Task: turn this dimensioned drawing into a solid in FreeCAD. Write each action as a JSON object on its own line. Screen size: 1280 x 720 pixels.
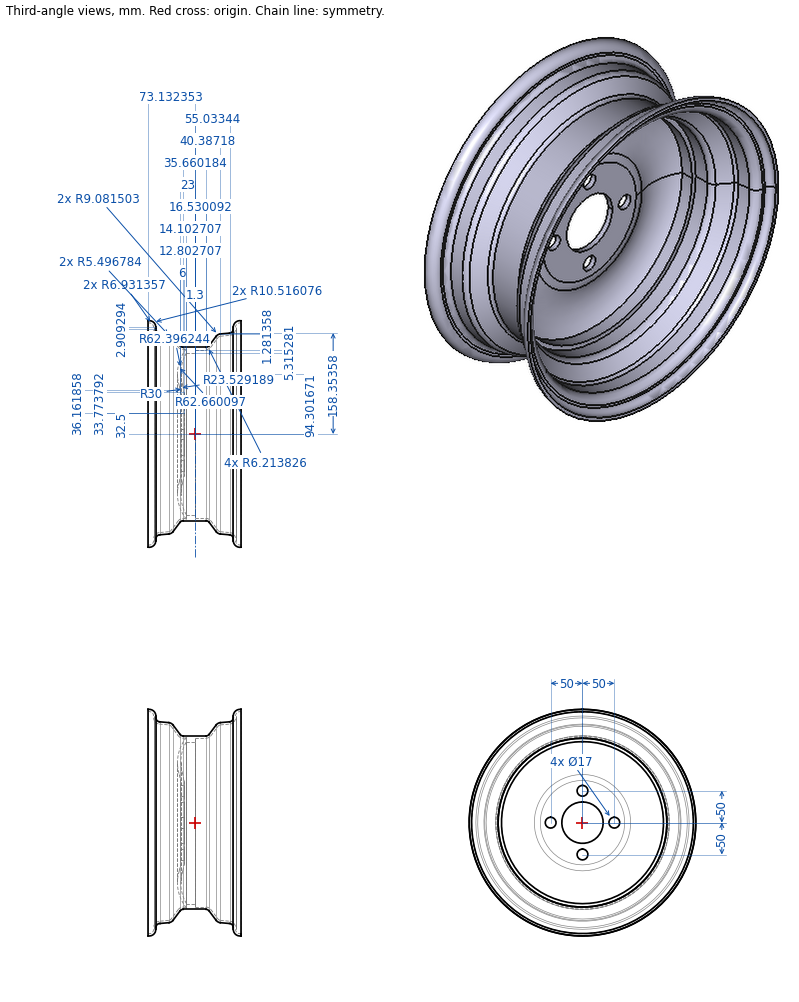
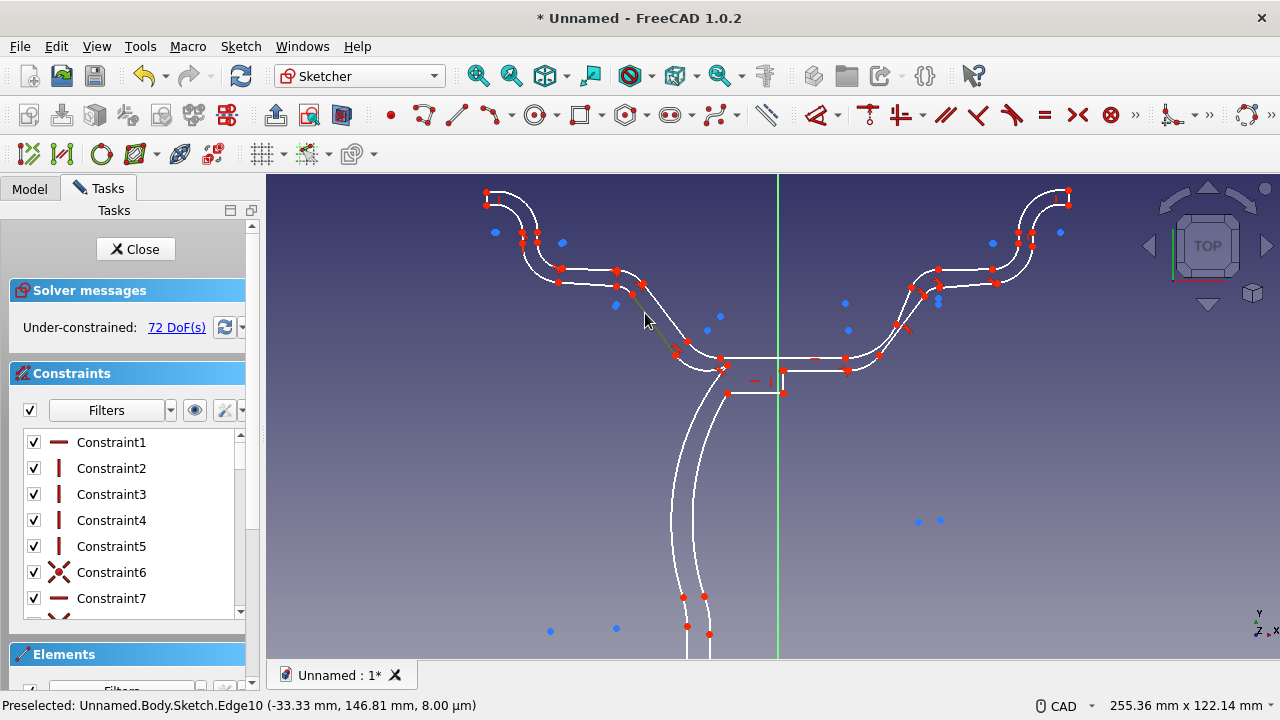
{"action": "left_click", "coordinate": [689, 366]}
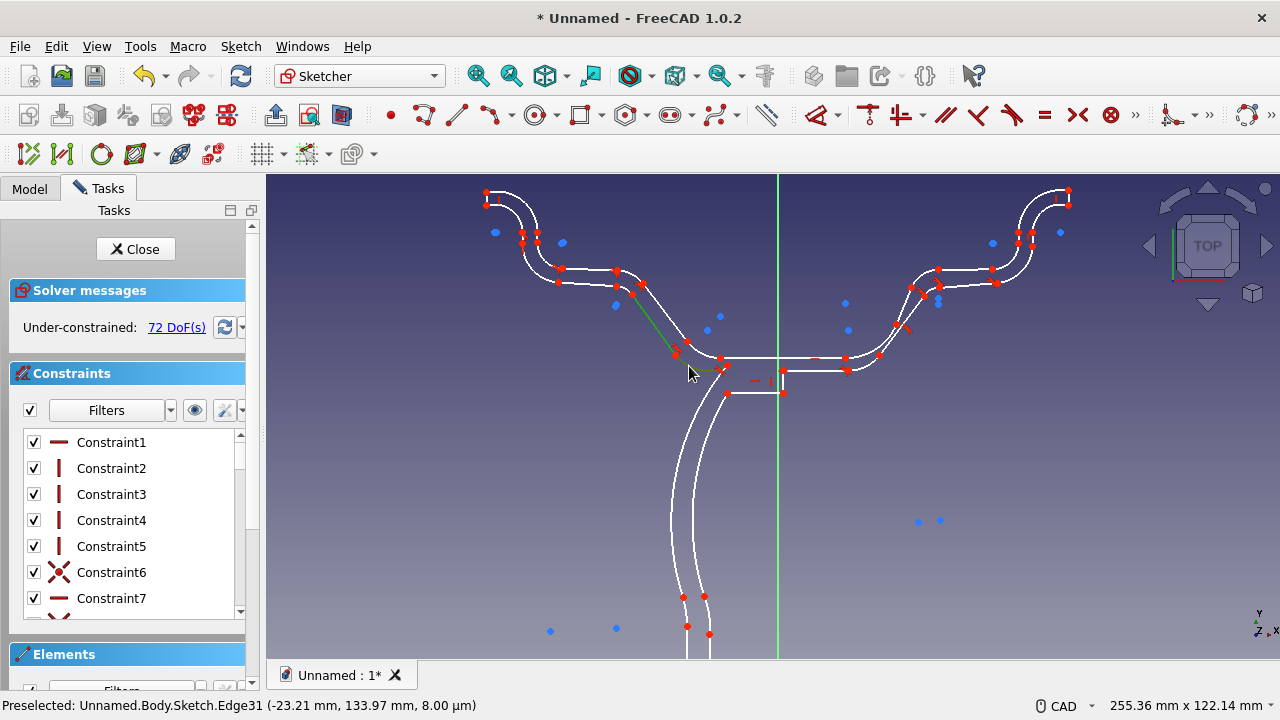
{"action": "key", "text": "t"}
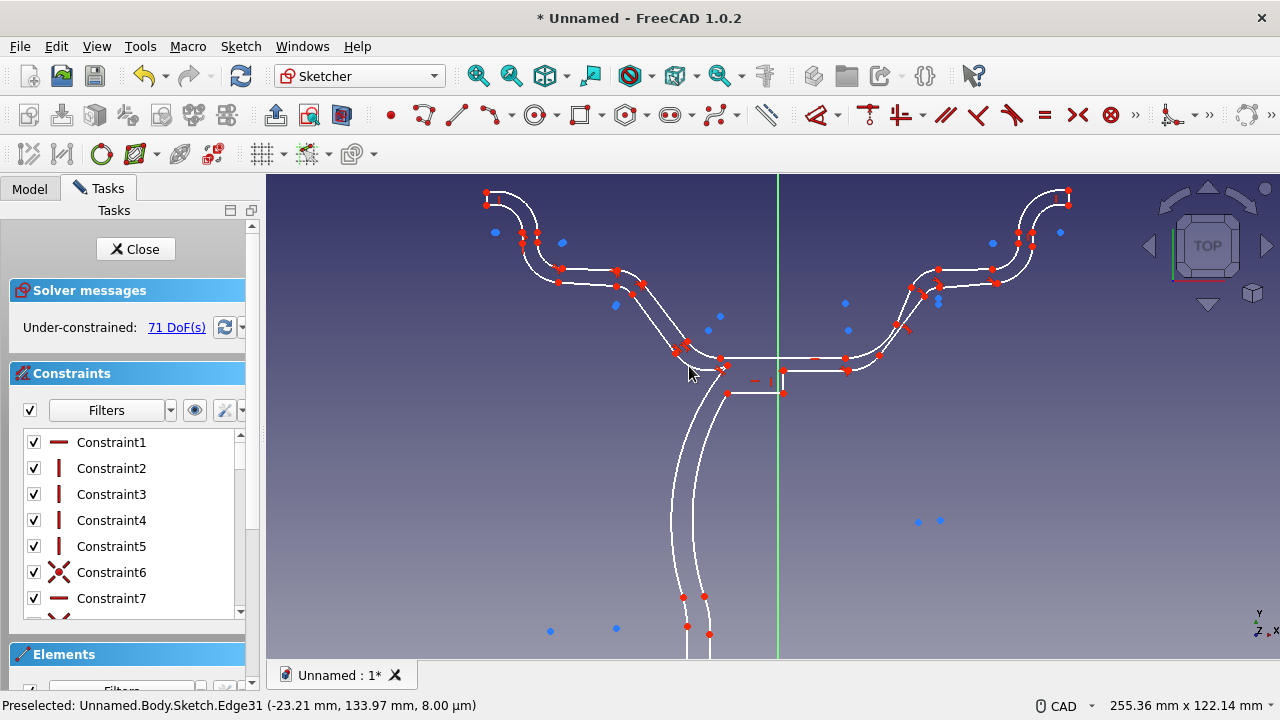
{"action": "scroll", "coordinate": [645, 313], "scroll_direction": "down", "scroll_amount": 4}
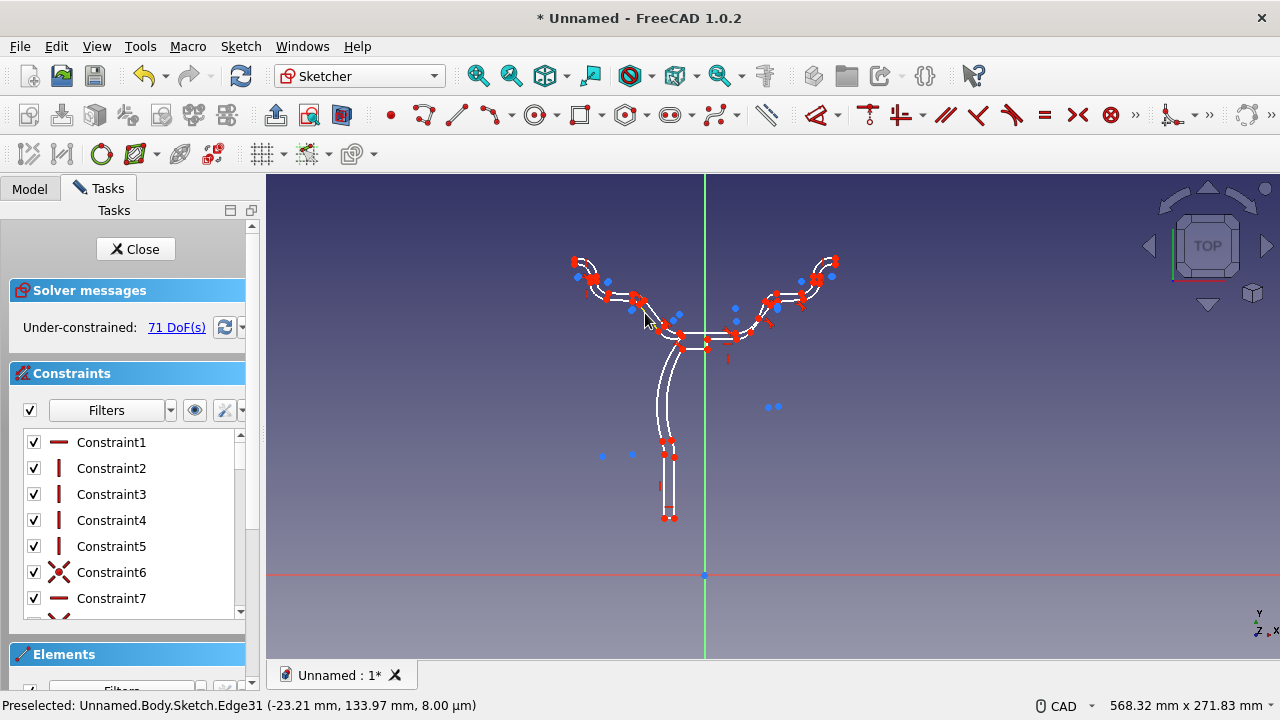
{"action": "scroll", "coordinate": [664, 473], "scroll_direction": "up", "scroll_amount": 2}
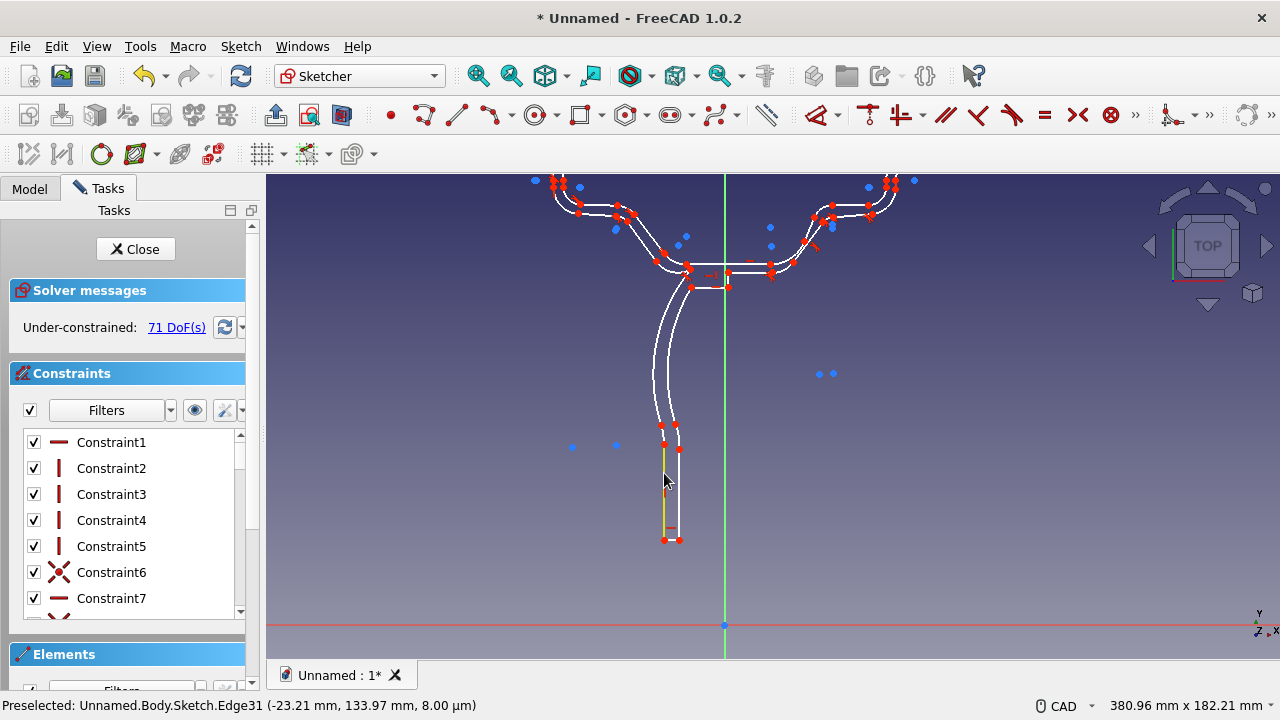
{"action": "left_click", "coordinate": [664, 473]}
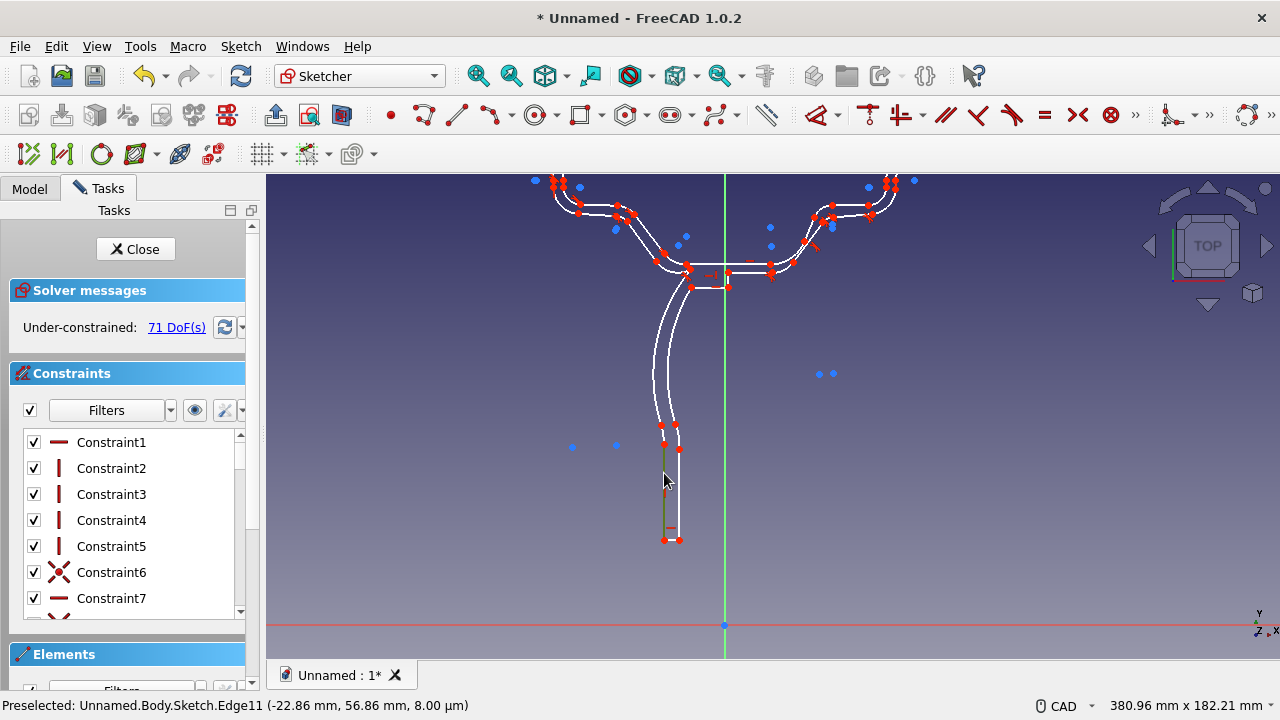
{"action": "scroll", "coordinate": [663, 435], "scroll_direction": "up", "scroll_amount": 2}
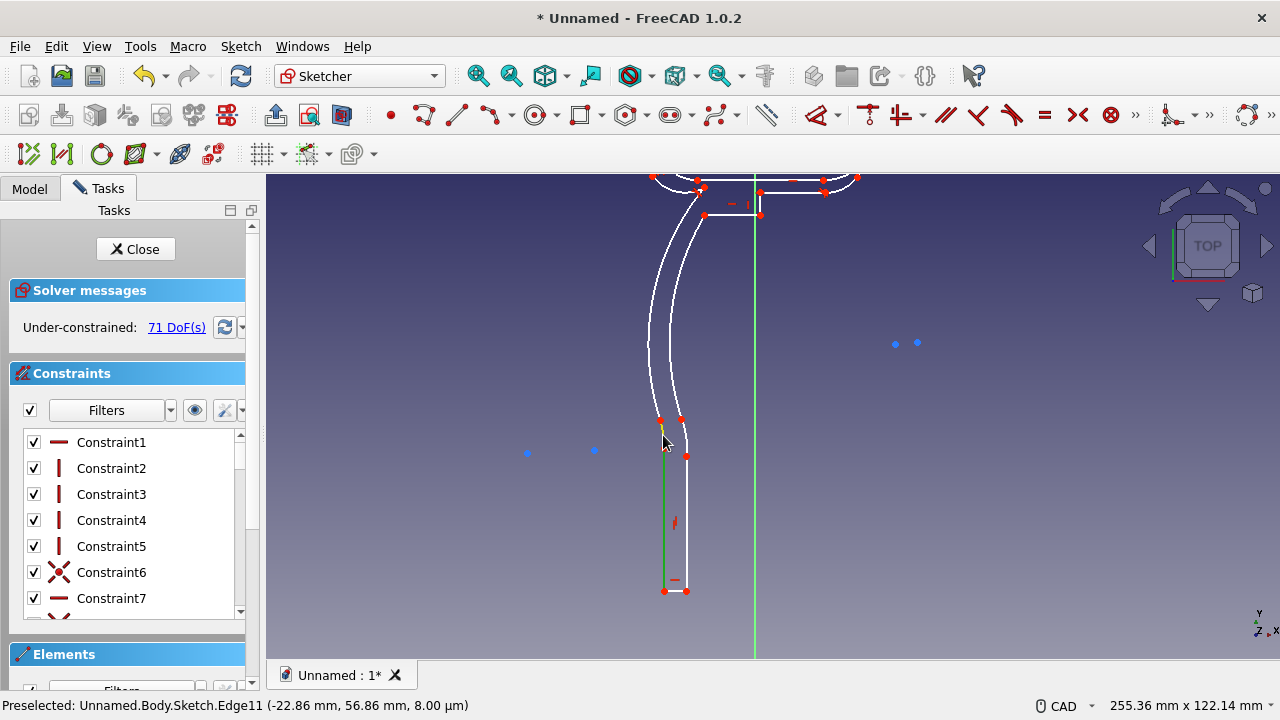
{"action": "left_click", "coordinate": [663, 434]}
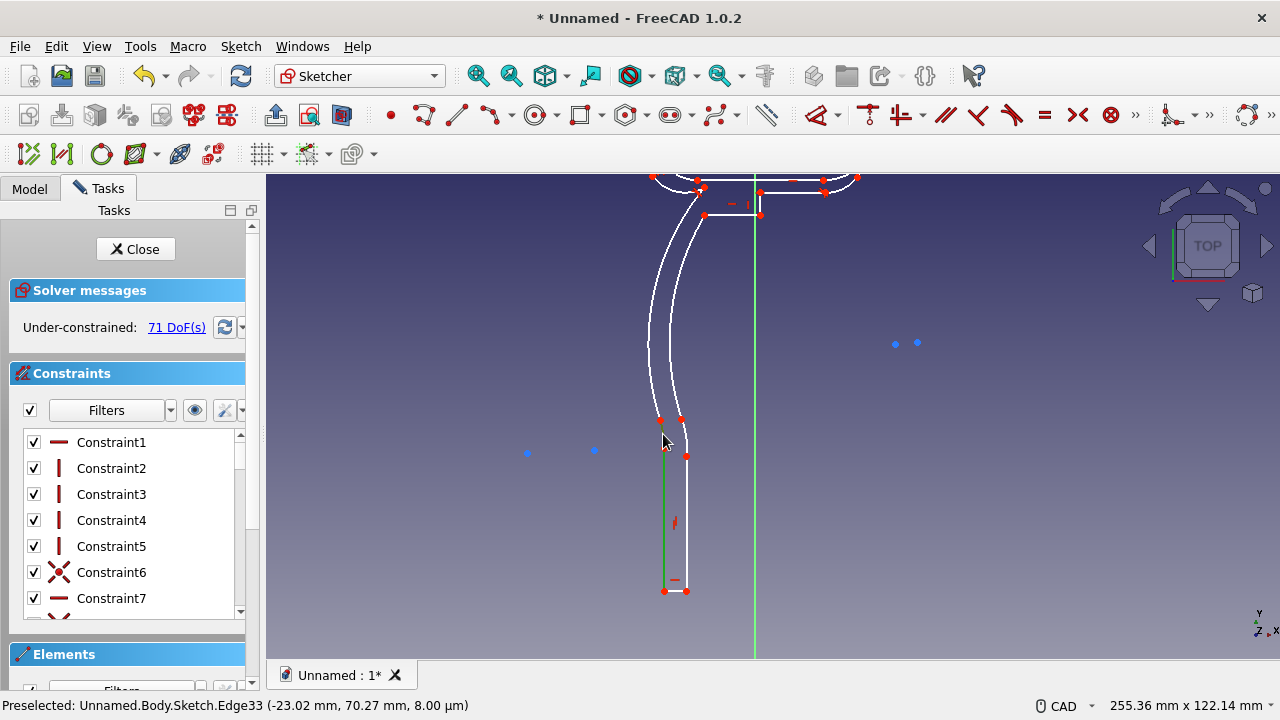
{"action": "left_click", "coordinate": [1012, 116]}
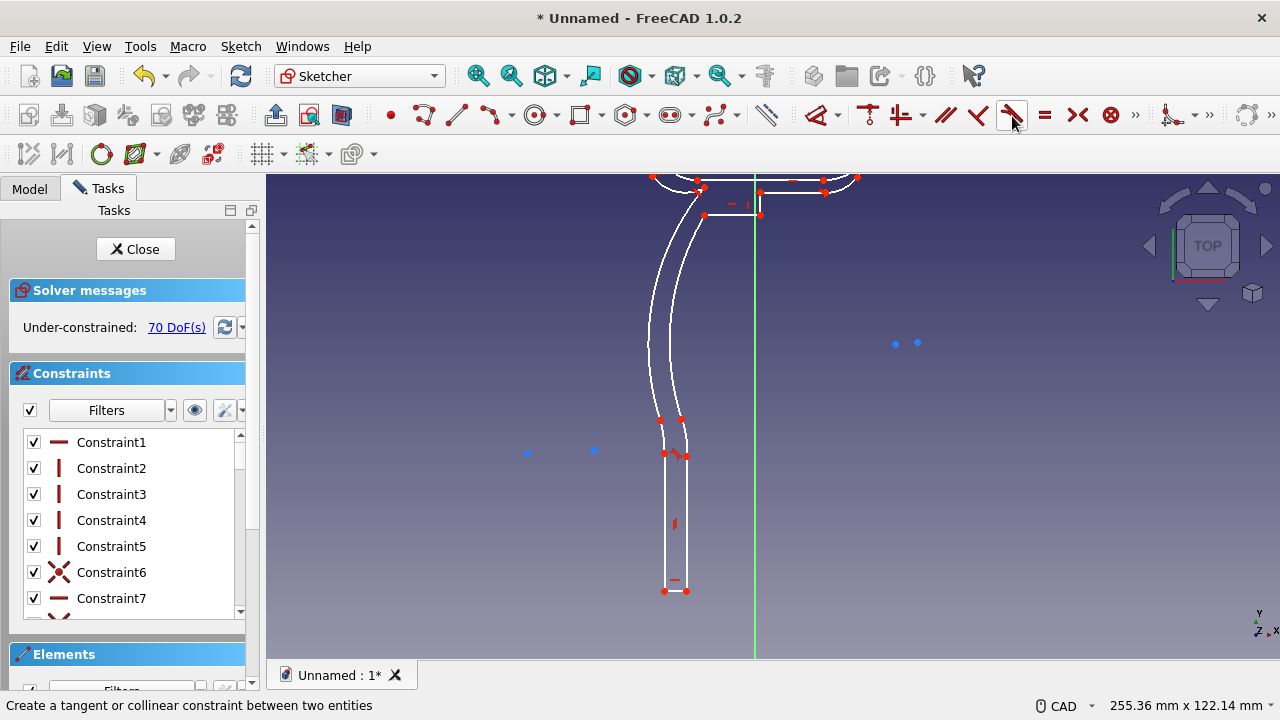
{"action": "left_click", "coordinate": [687, 551]}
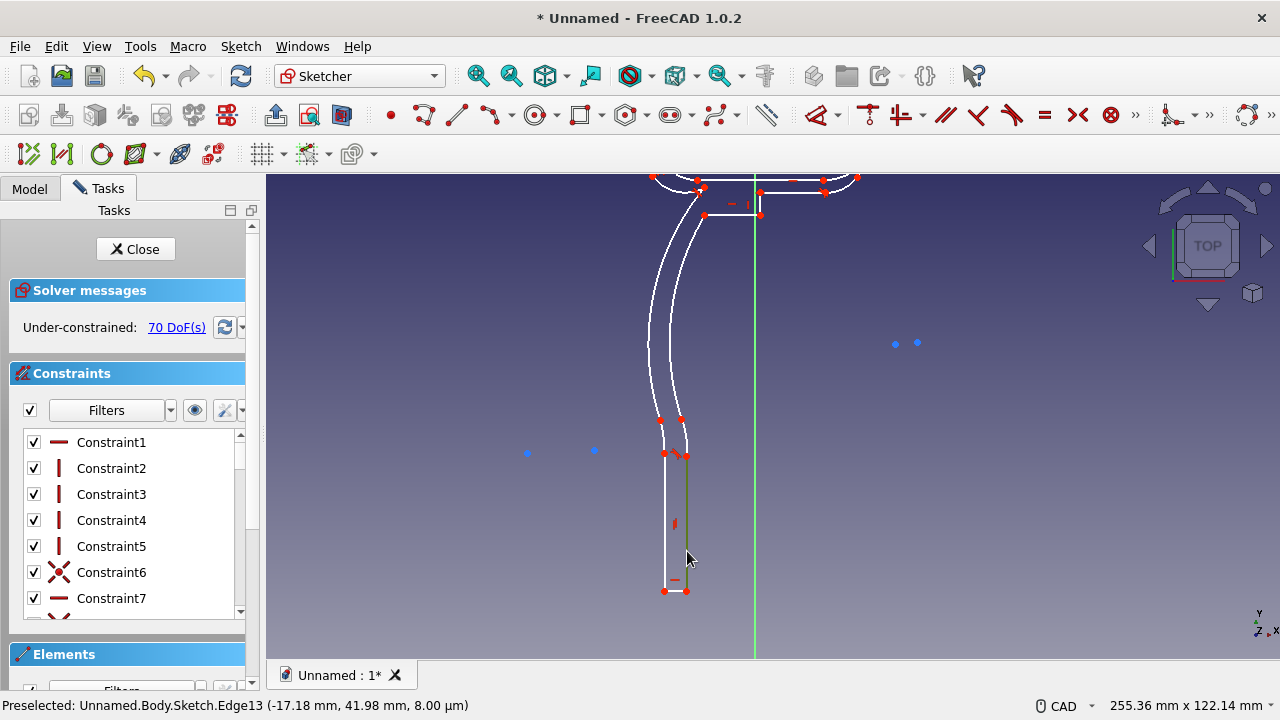
{"action": "left_click", "coordinate": [687, 445]}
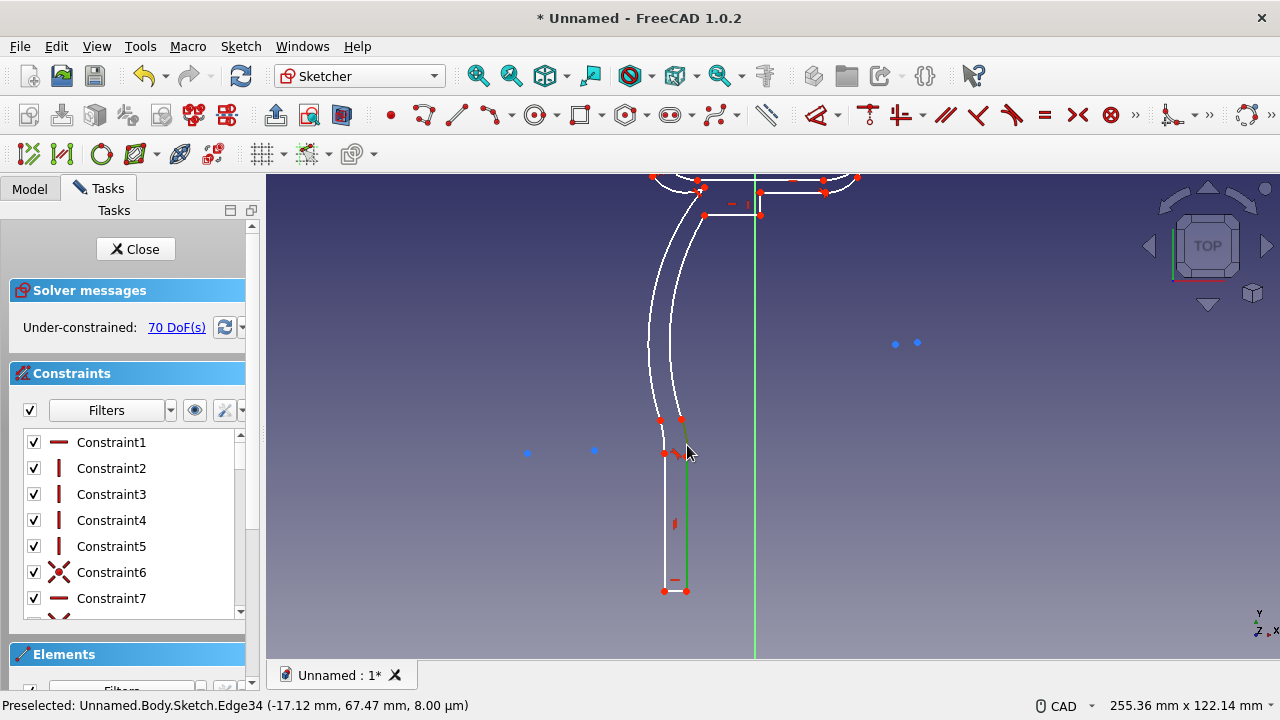
{"action": "key", "text": "t"}